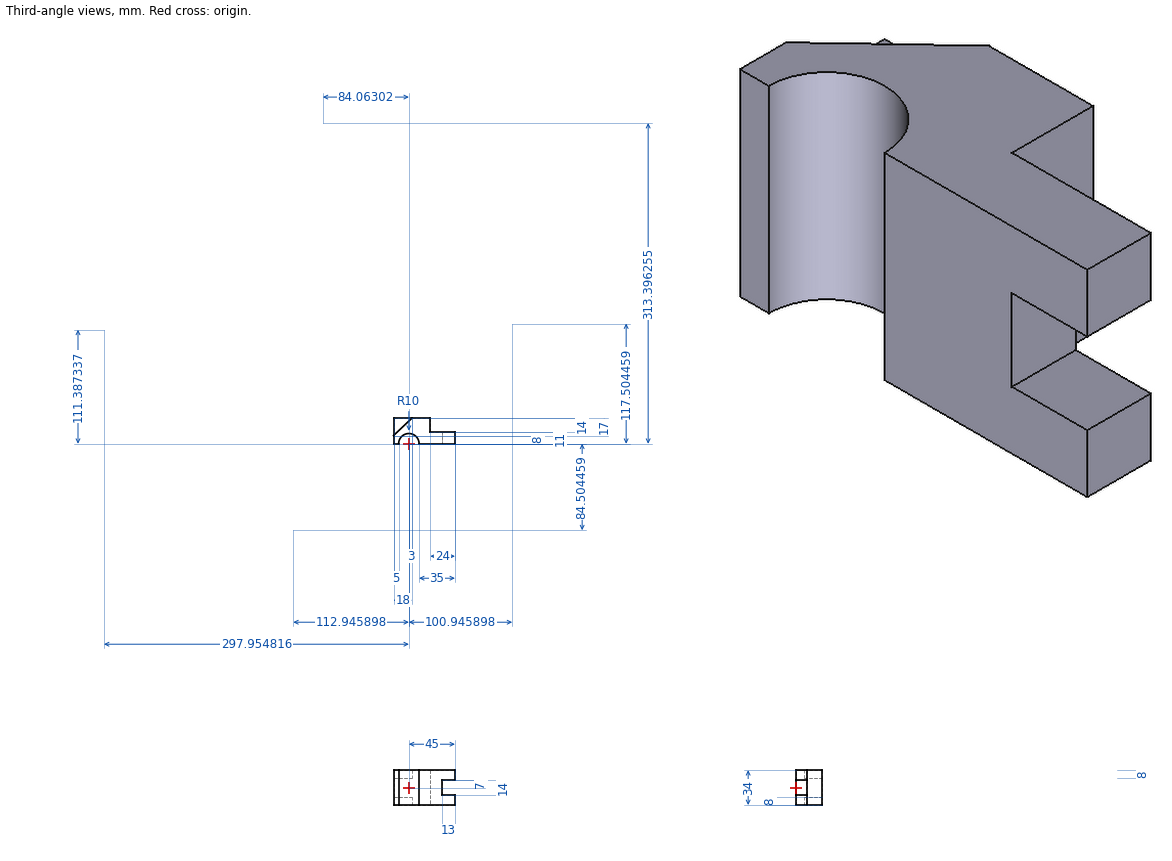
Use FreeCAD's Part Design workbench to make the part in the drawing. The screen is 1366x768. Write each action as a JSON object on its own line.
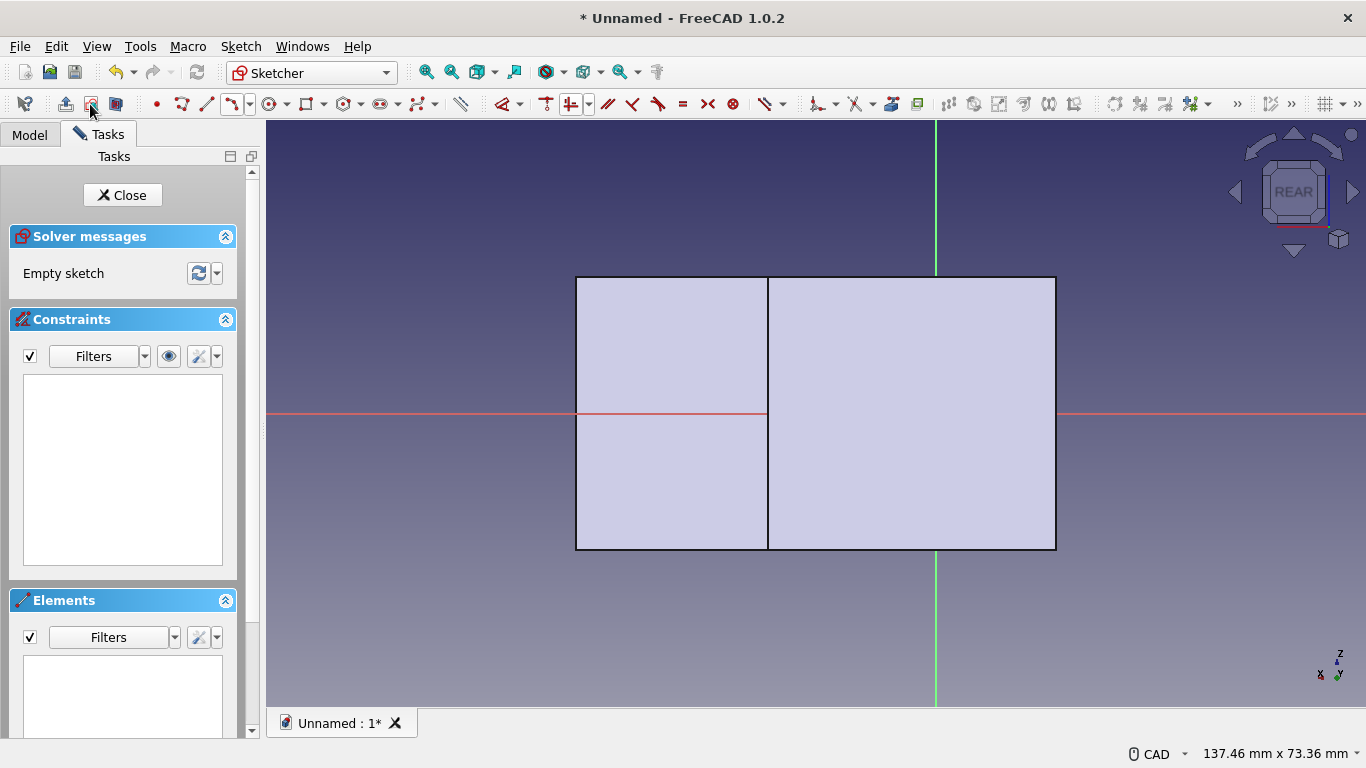
{"action": "scroll", "coordinate": [576, 414], "scroll_direction": "up", "scroll_amount": 6}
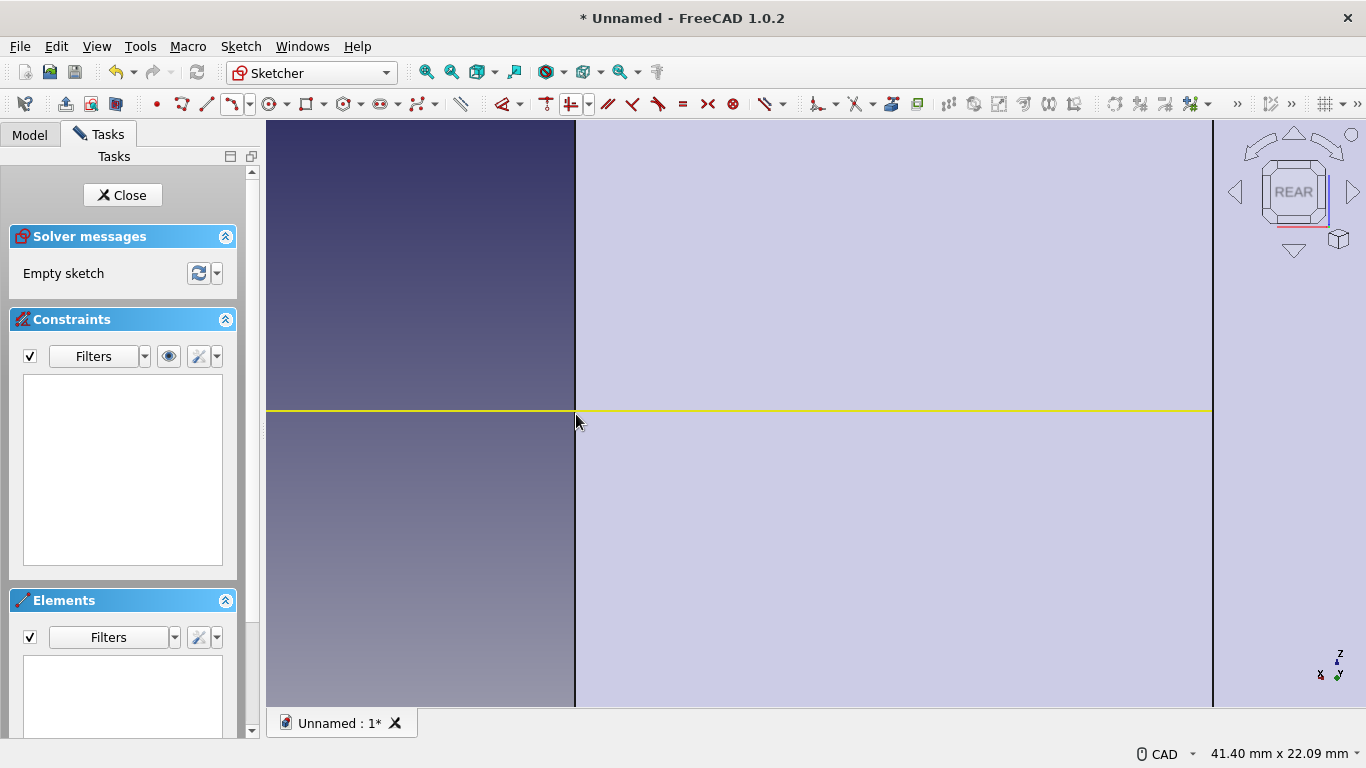
{"action": "left_click", "coordinate": [306, 104]}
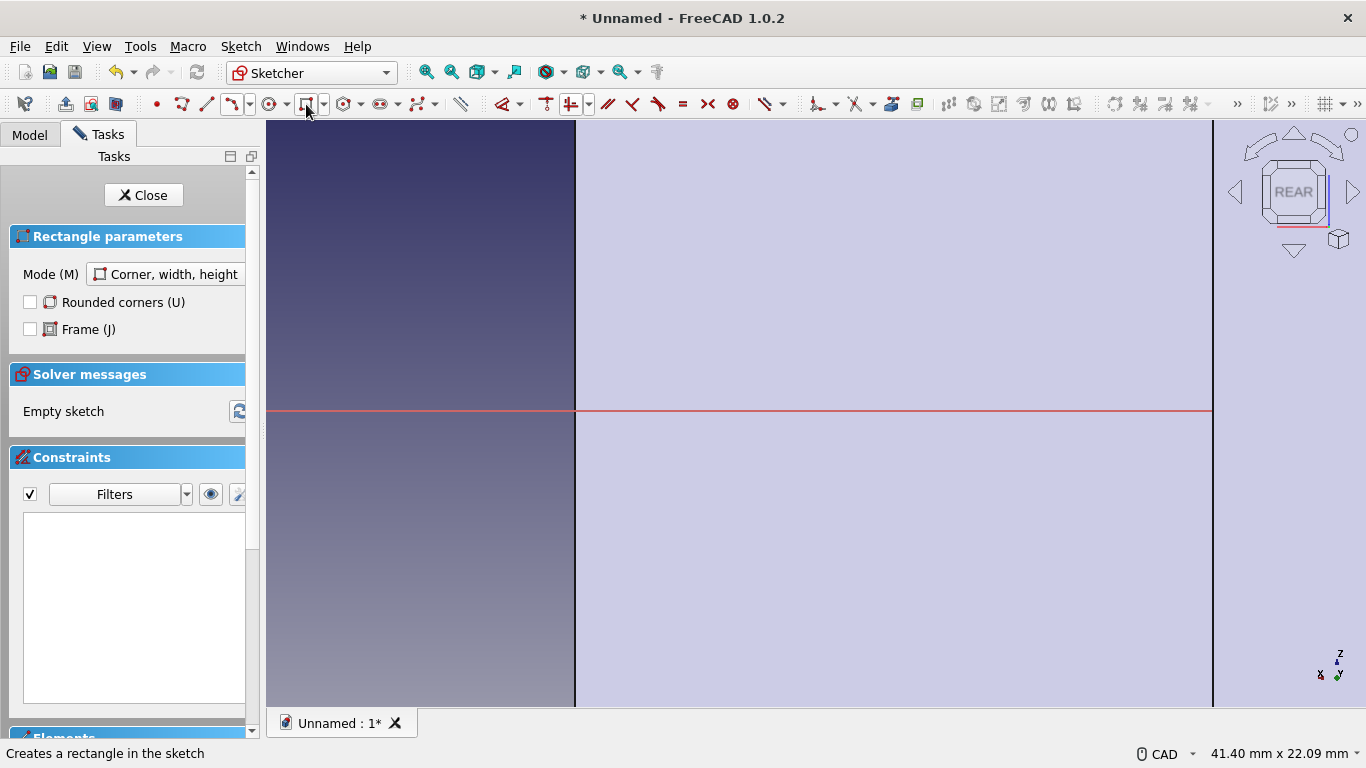
{"action": "left_click", "coordinate": [575, 225]}
{"action": "mouse_move", "coordinate": [921, 597]}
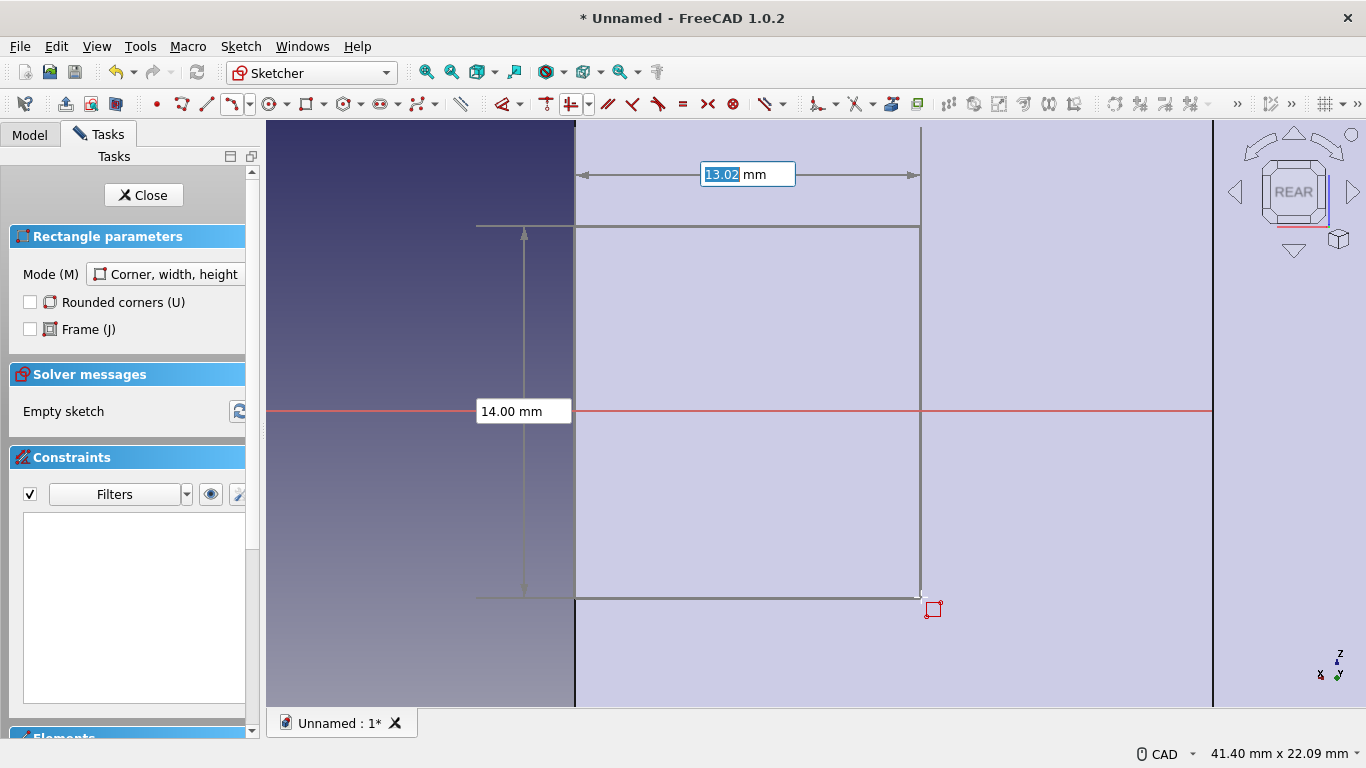
{"action": "type", "text": "13"}
{"action": "key", "text": "Tab"}
{"action": "type", "text": "14"}
{"action": "key", "text": "Return"}
{"action": "key", "text": "Escape"}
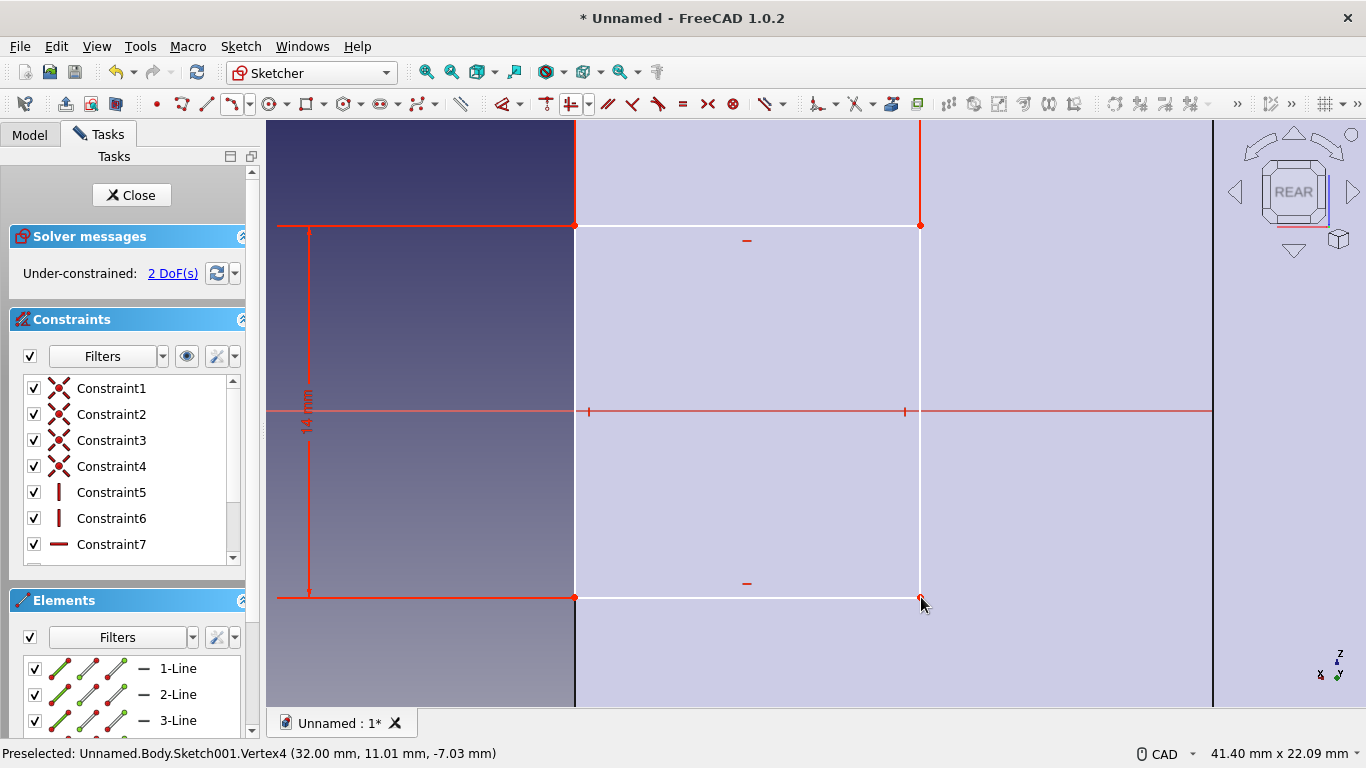
{"action": "left_click", "coordinate": [502, 104]}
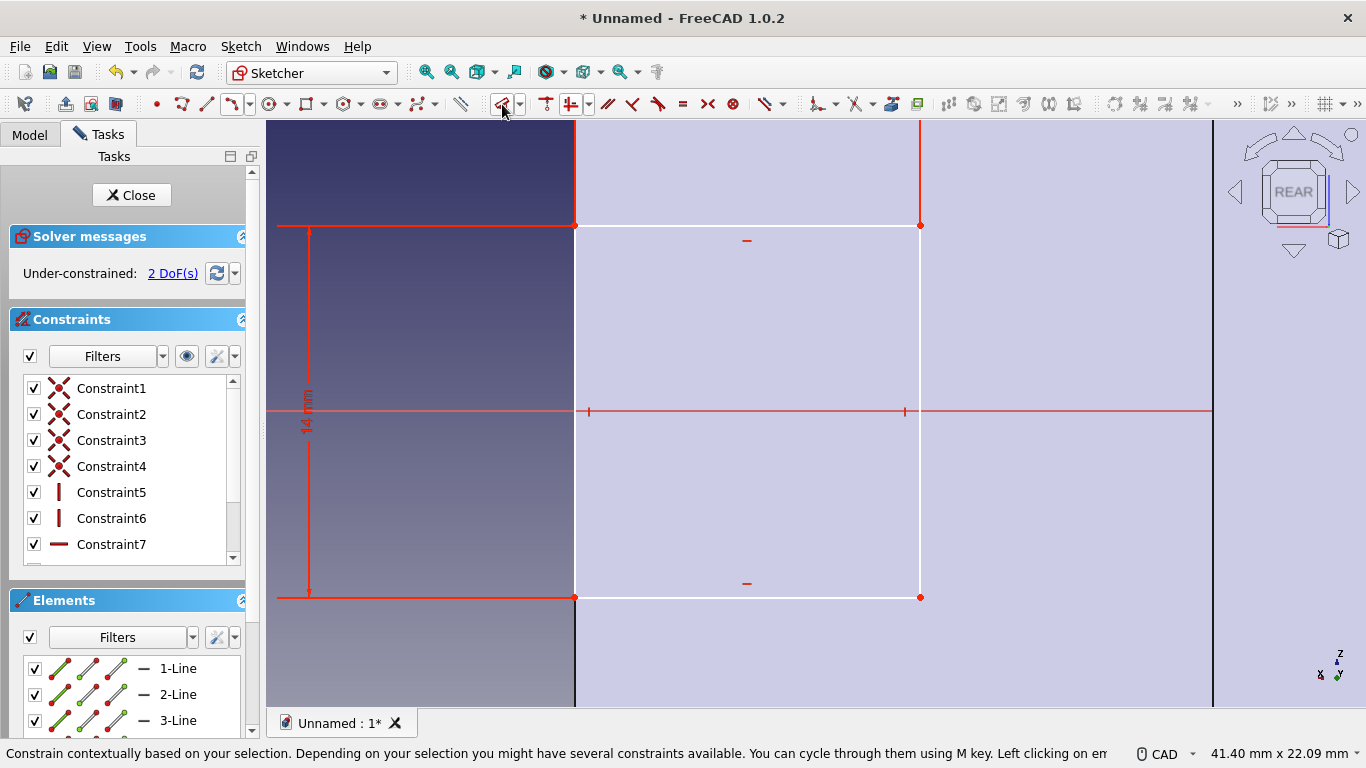
{"action": "left_click", "coordinate": [575, 226]}
{"action": "left_click", "coordinate": [541, 319]}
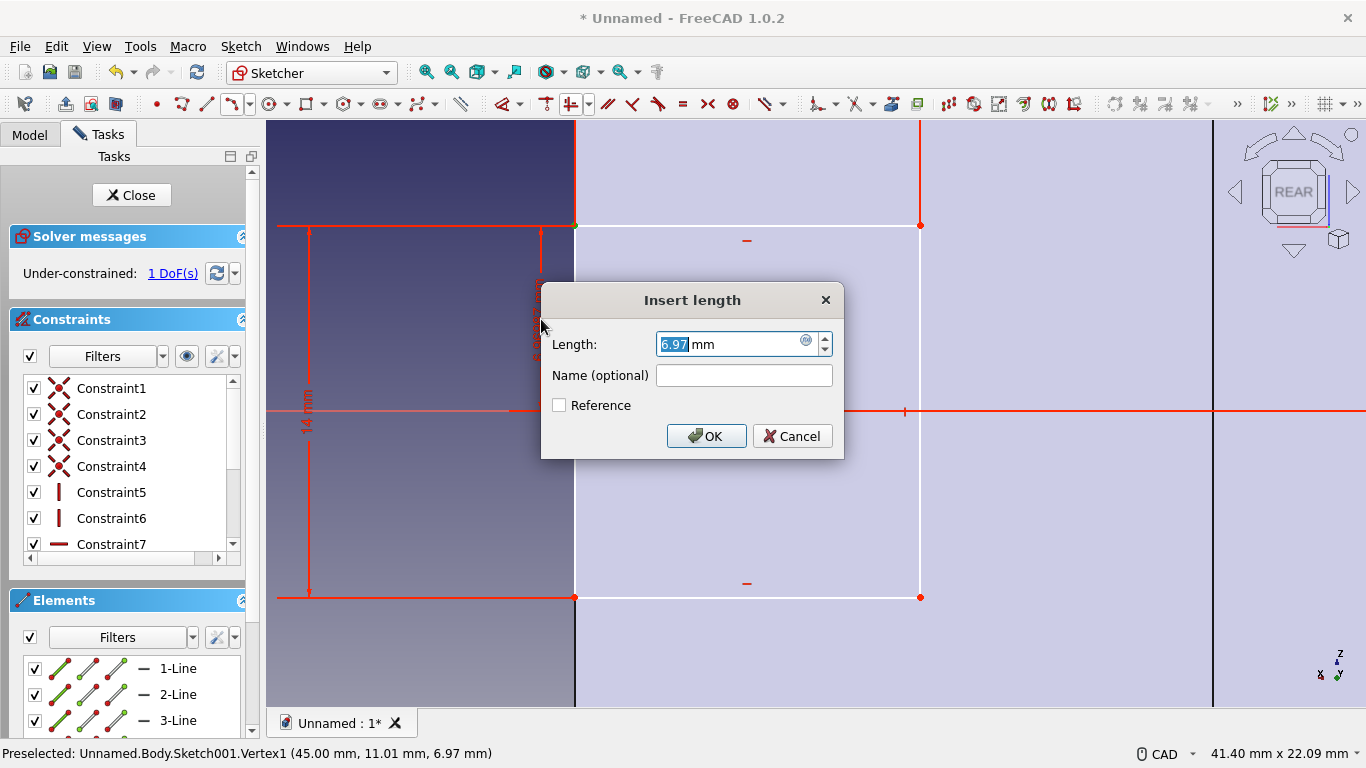
{"action": "type", "text": "7"}
{"action": "key", "text": "Return"}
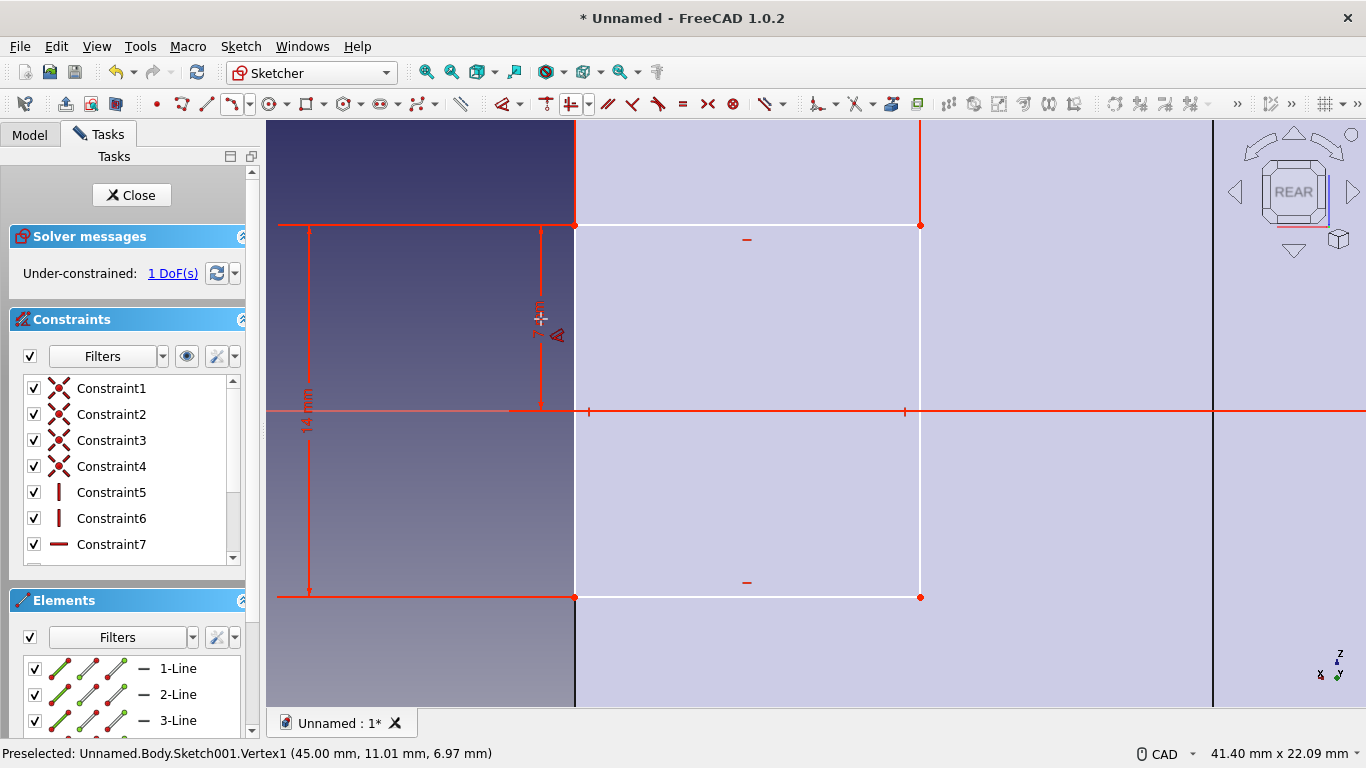
{"action": "left_click", "coordinate": [575, 225]}
{"action": "left_click", "coordinate": [888, 191]}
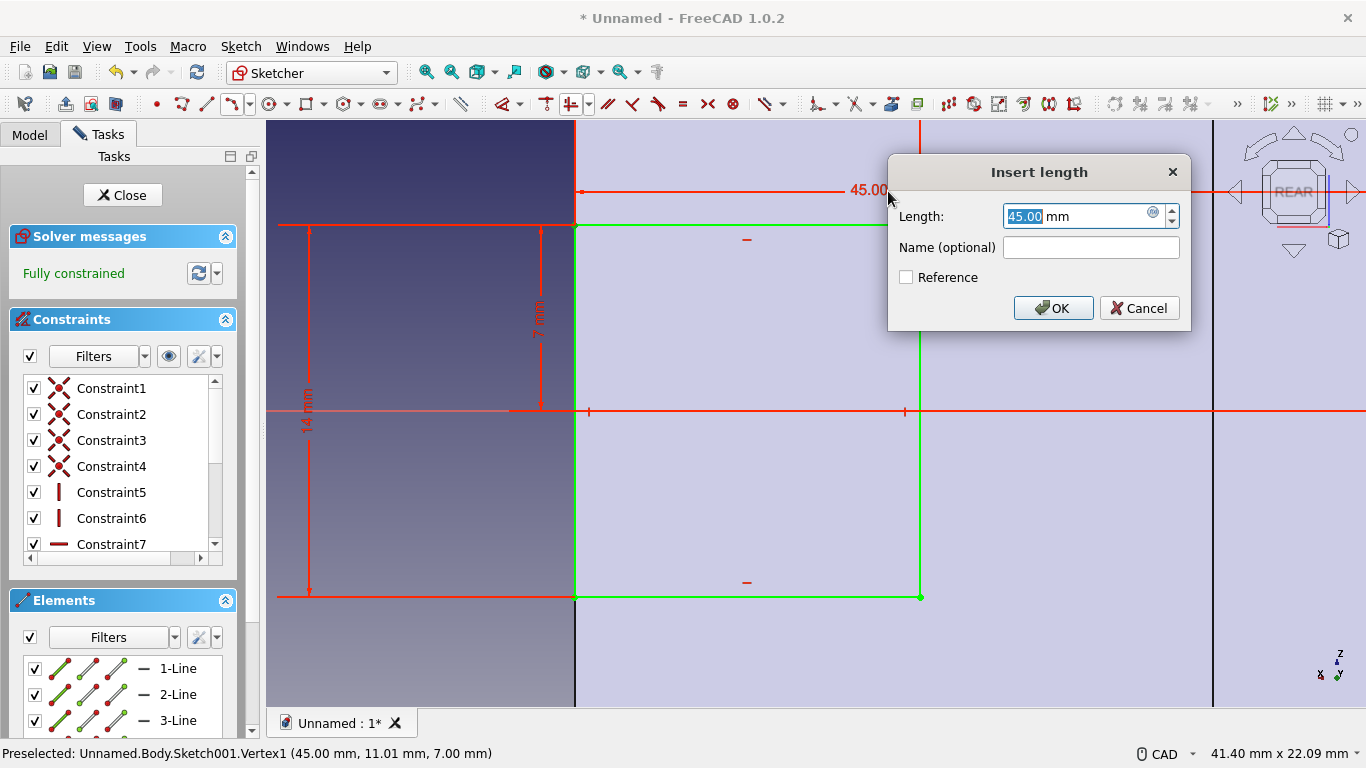
{"action": "type", "text": "45"}
{"action": "key", "text": "Return"}
{"action": "key", "text": "Escape"}